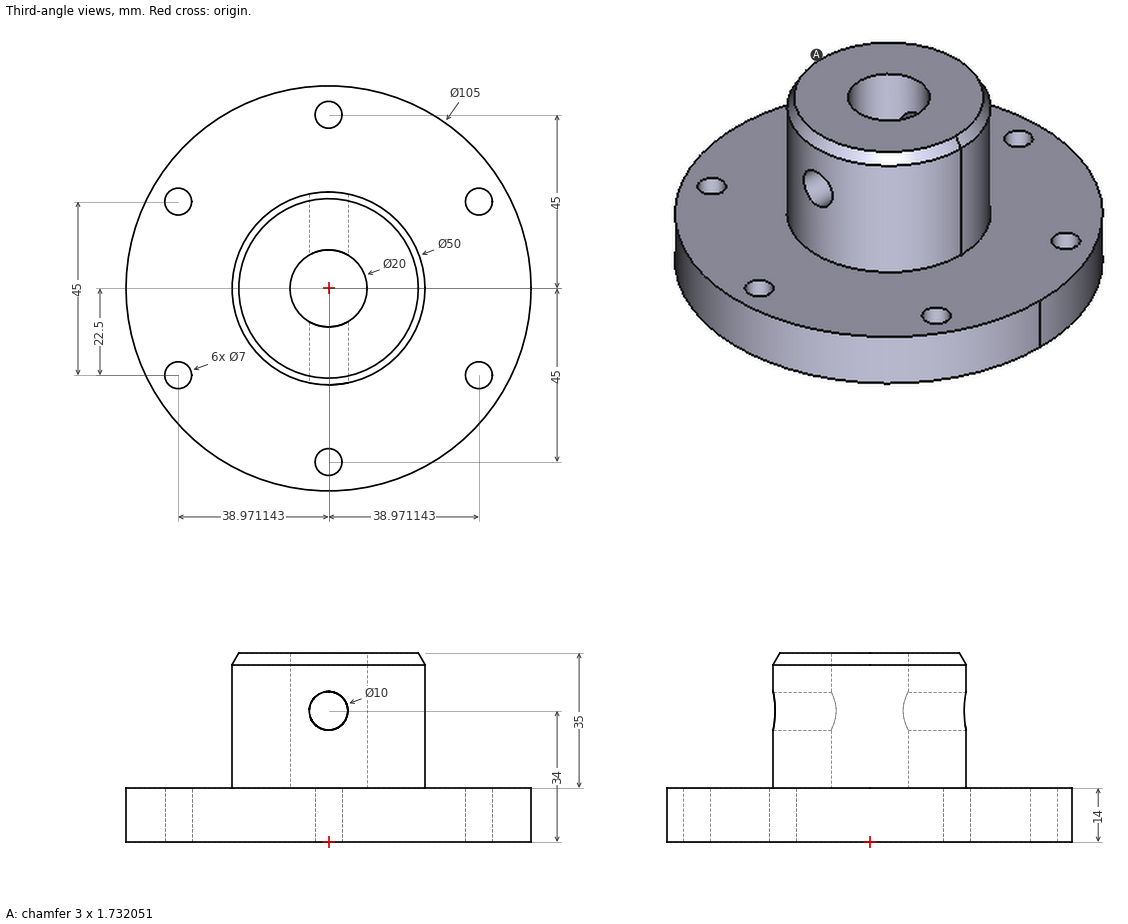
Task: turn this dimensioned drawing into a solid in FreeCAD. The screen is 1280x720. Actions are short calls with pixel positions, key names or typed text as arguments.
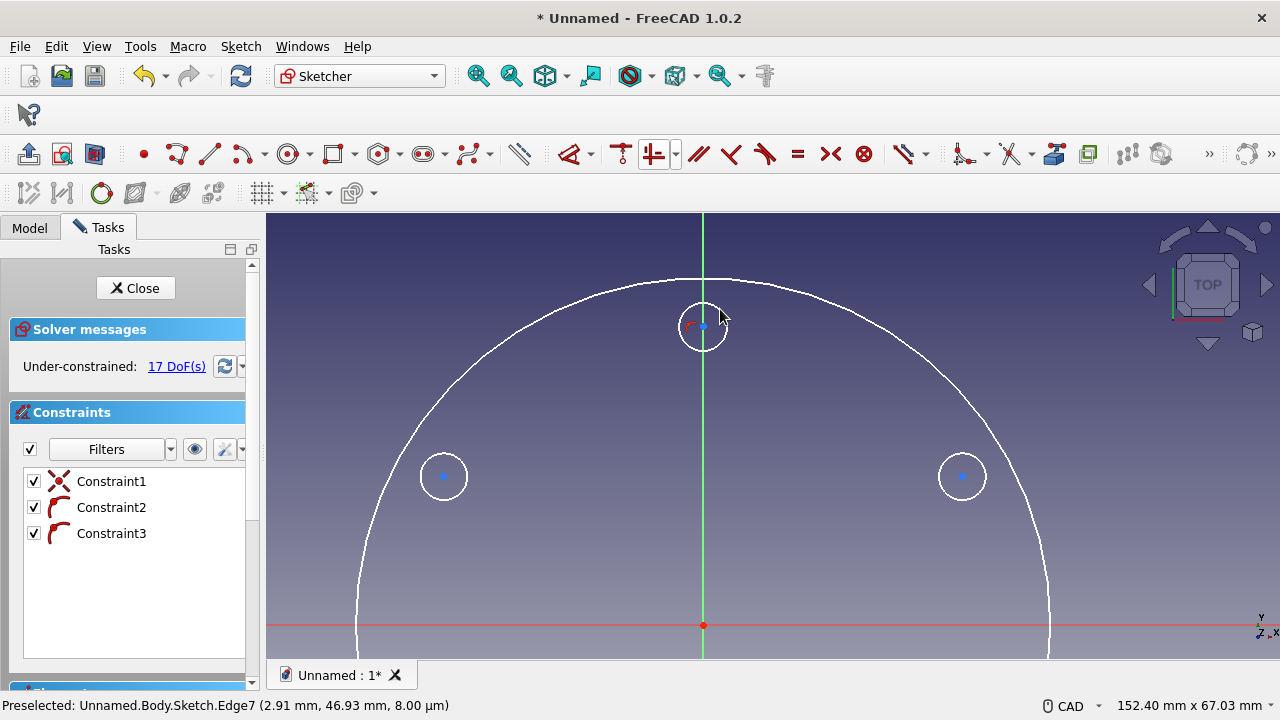
scroll(705, 326, down, 5)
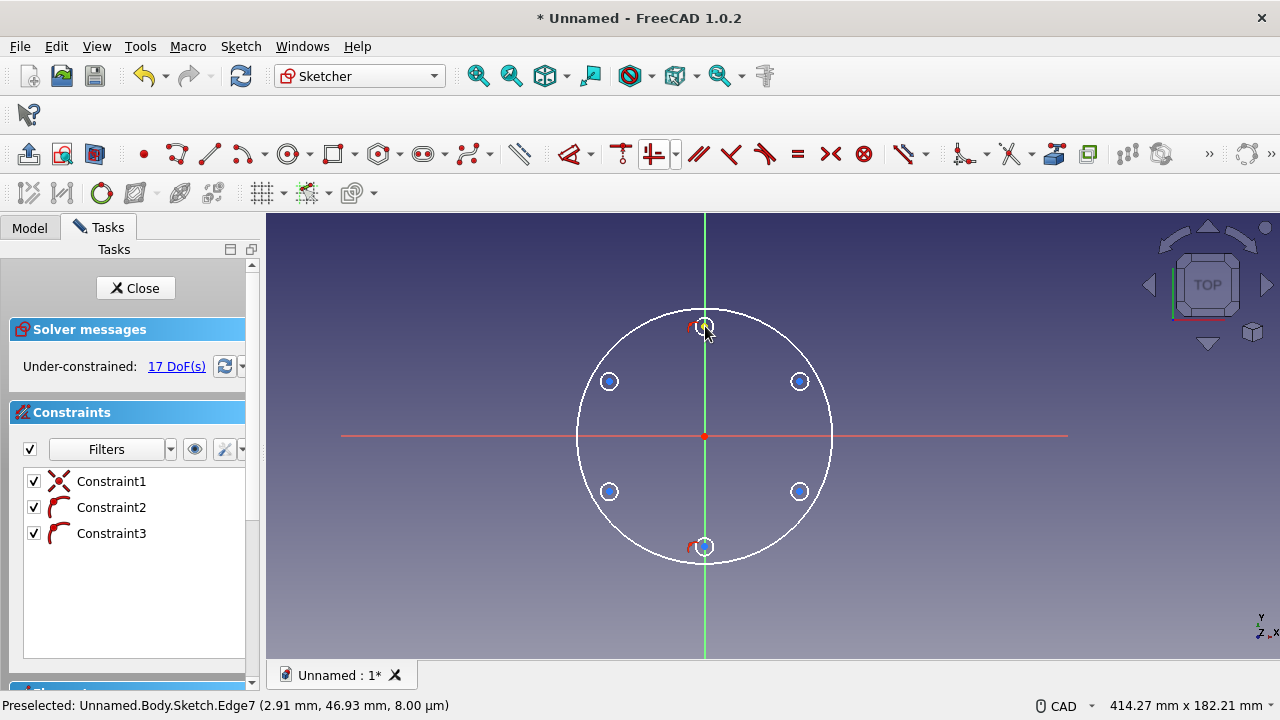
scroll(615, 486, up, 3)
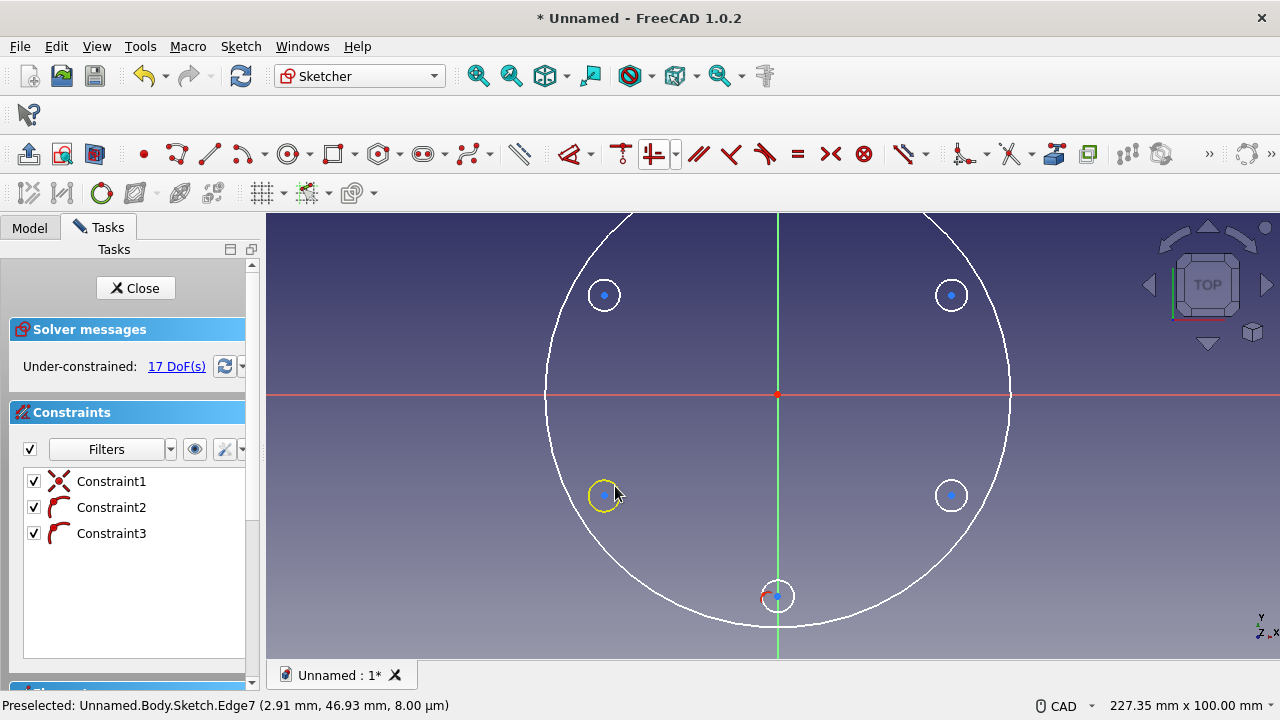
click(615, 485)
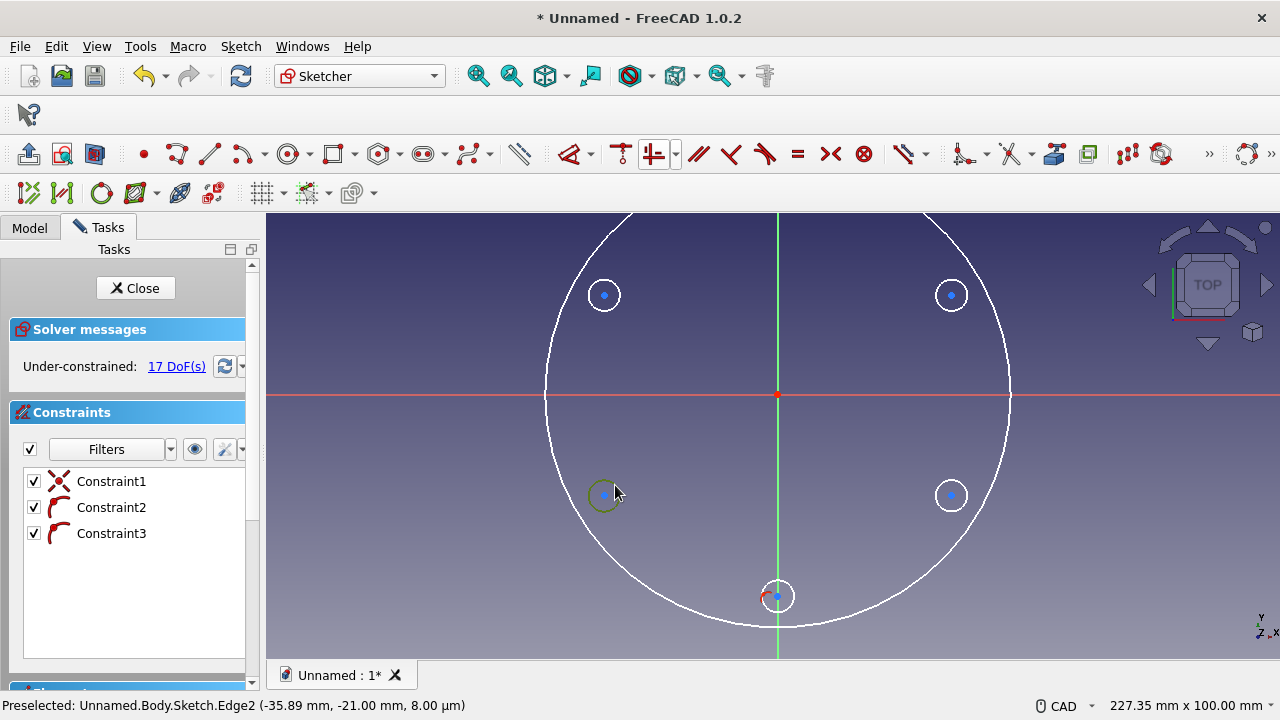
click(789, 585)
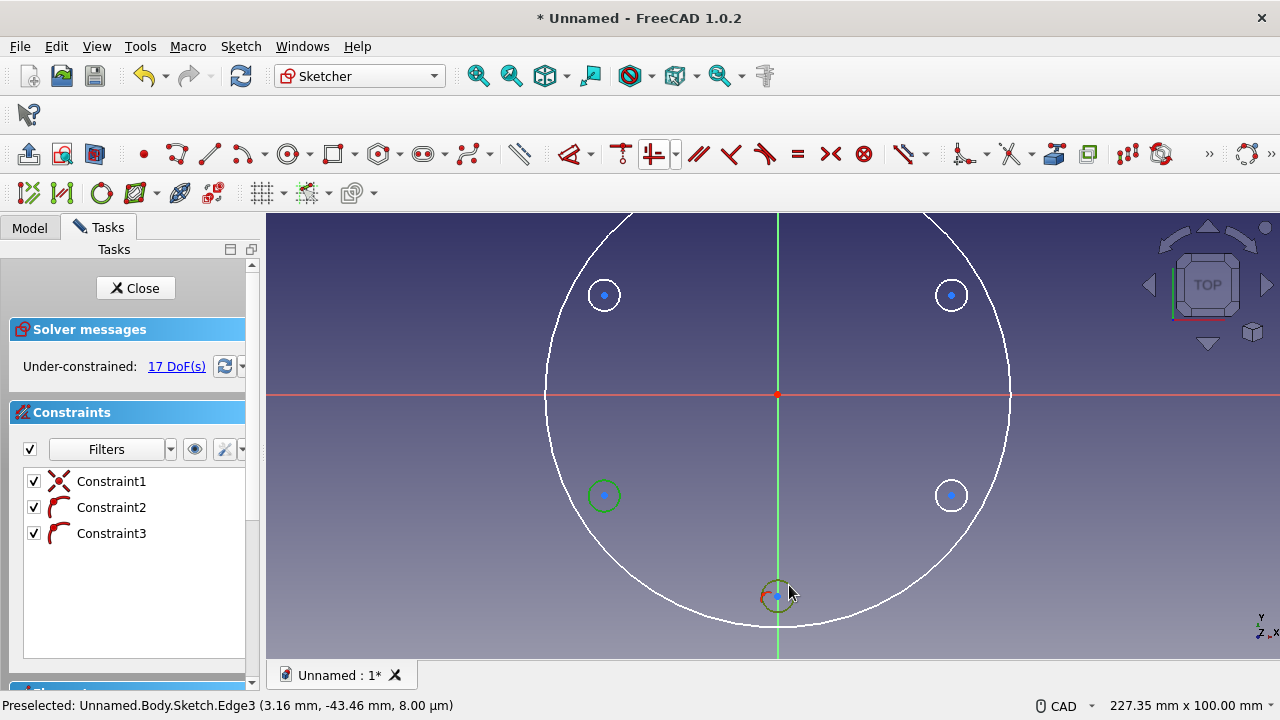
click(963, 485)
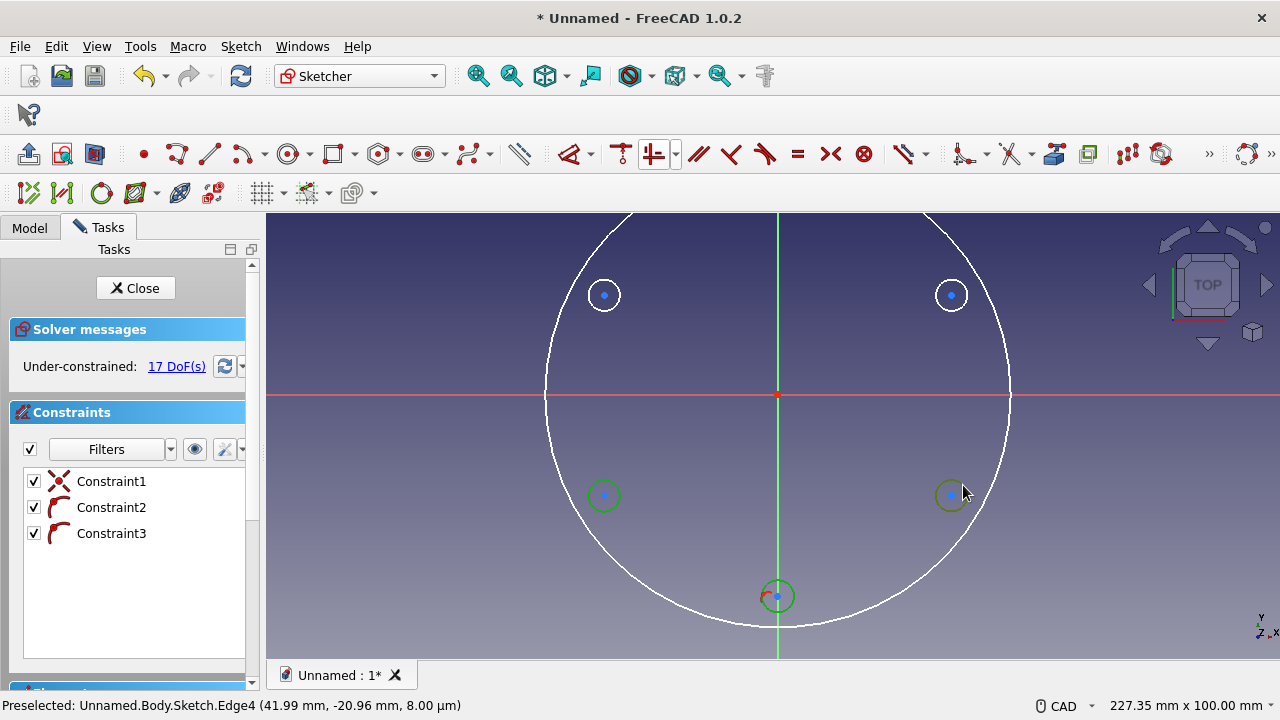
click(615, 284)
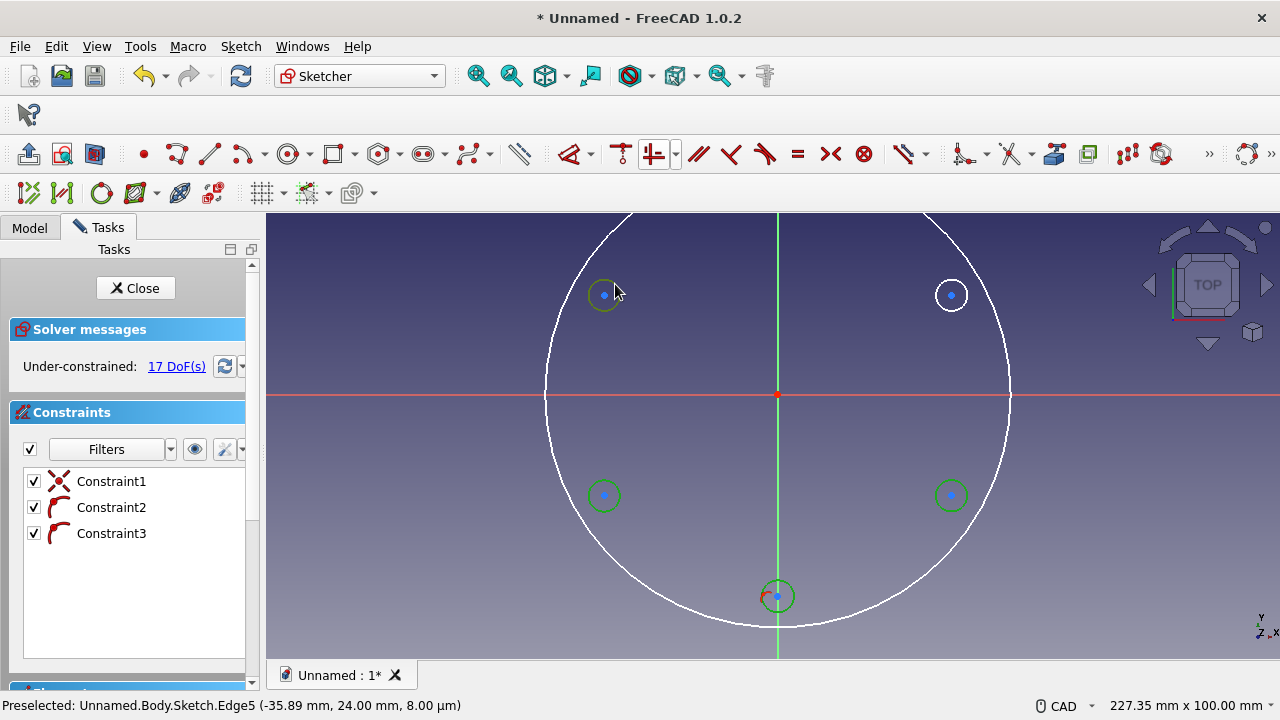
click(963, 284)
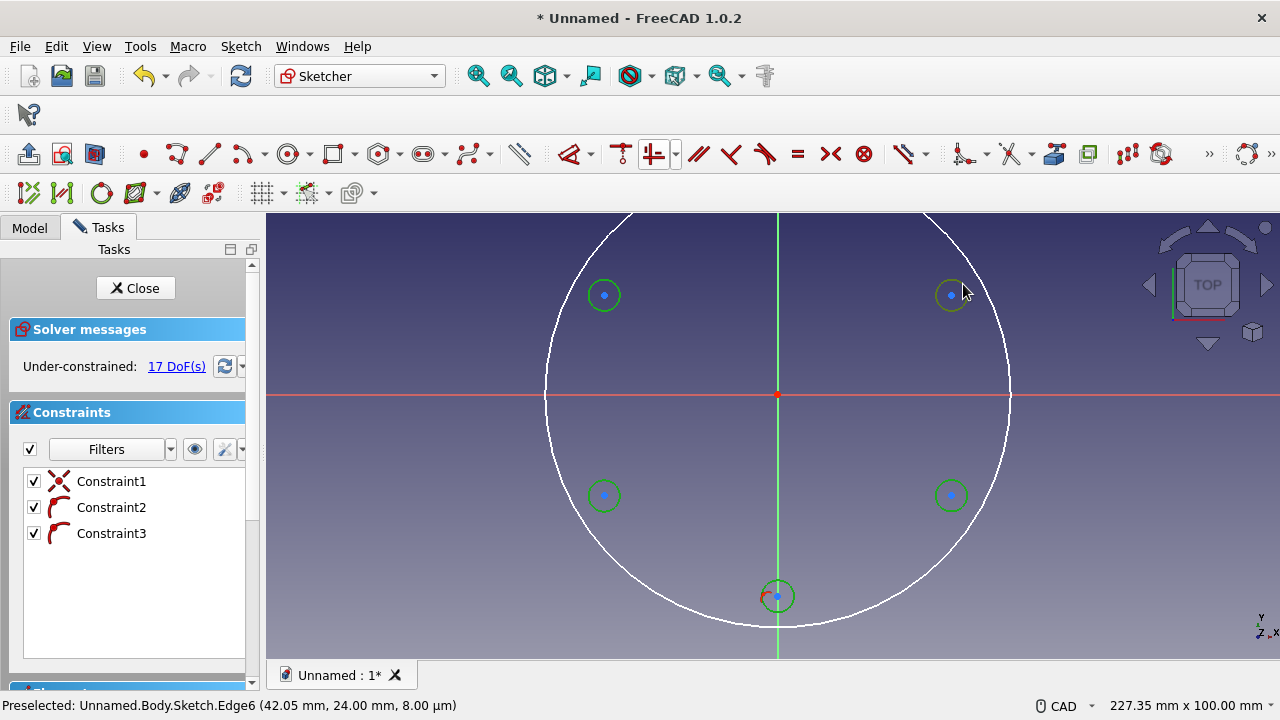
scroll(615, 486, down, 3)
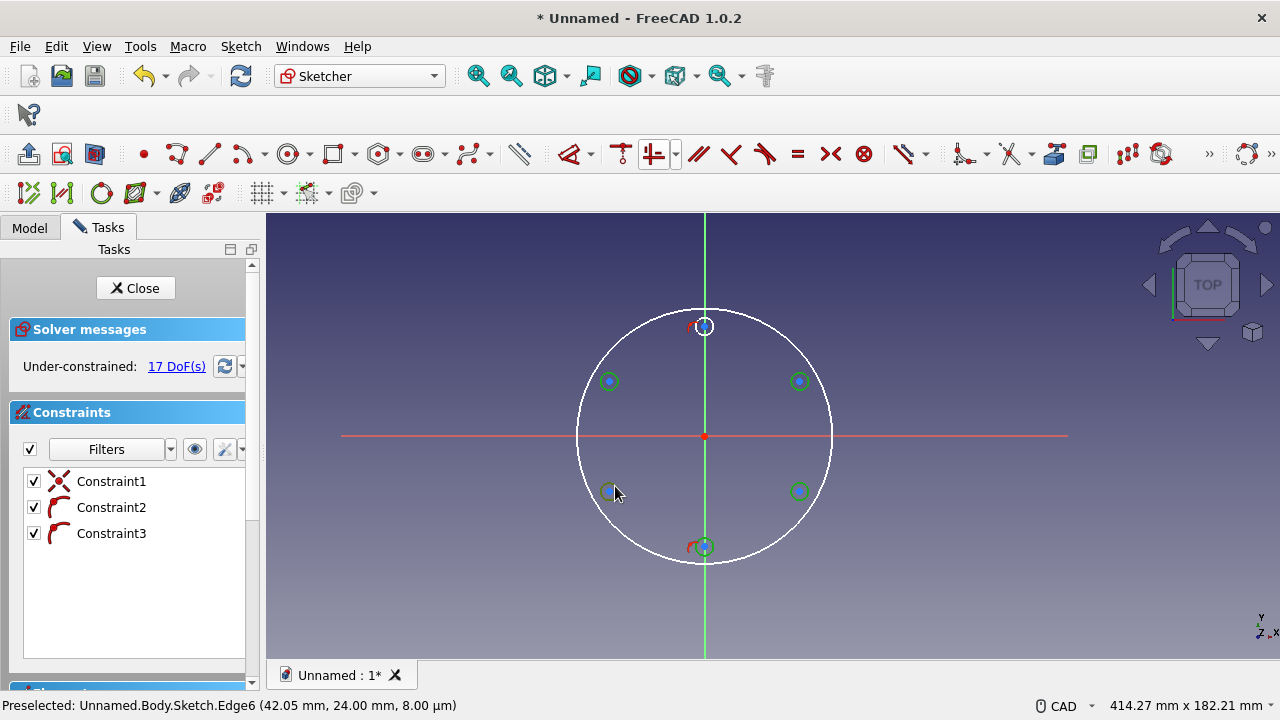
scroll(711, 320, up, 4)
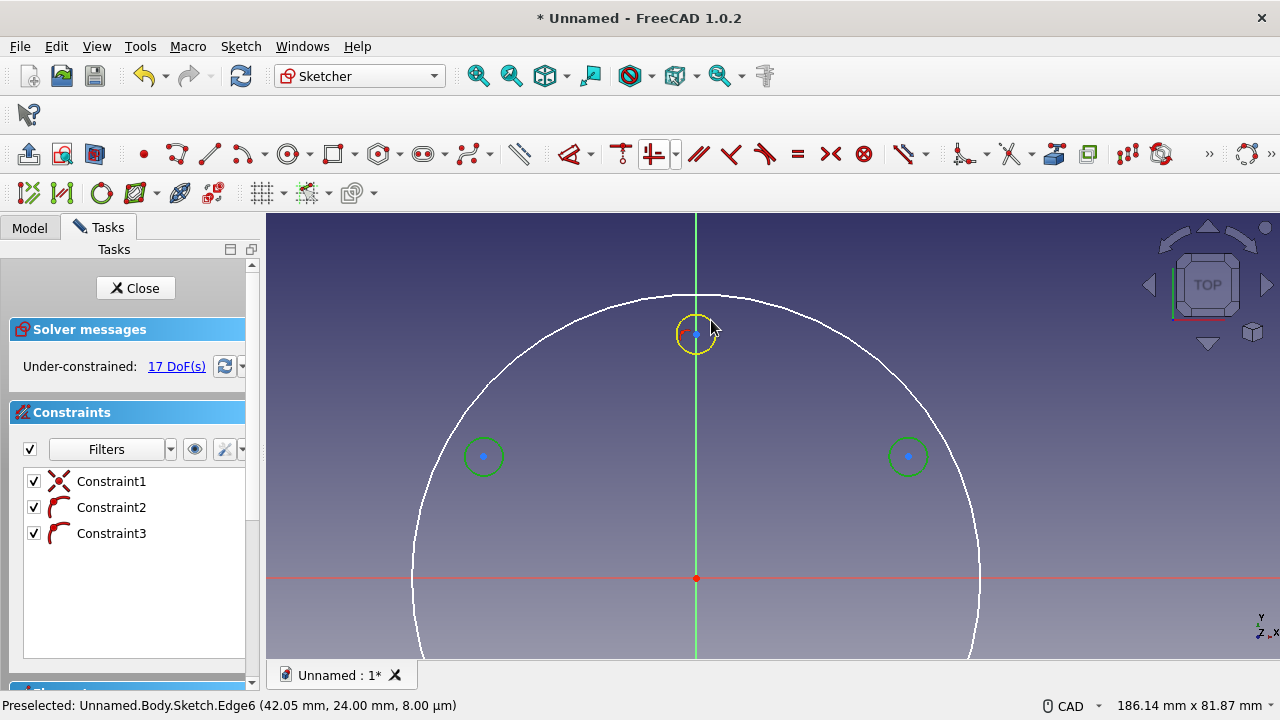
click(710, 320)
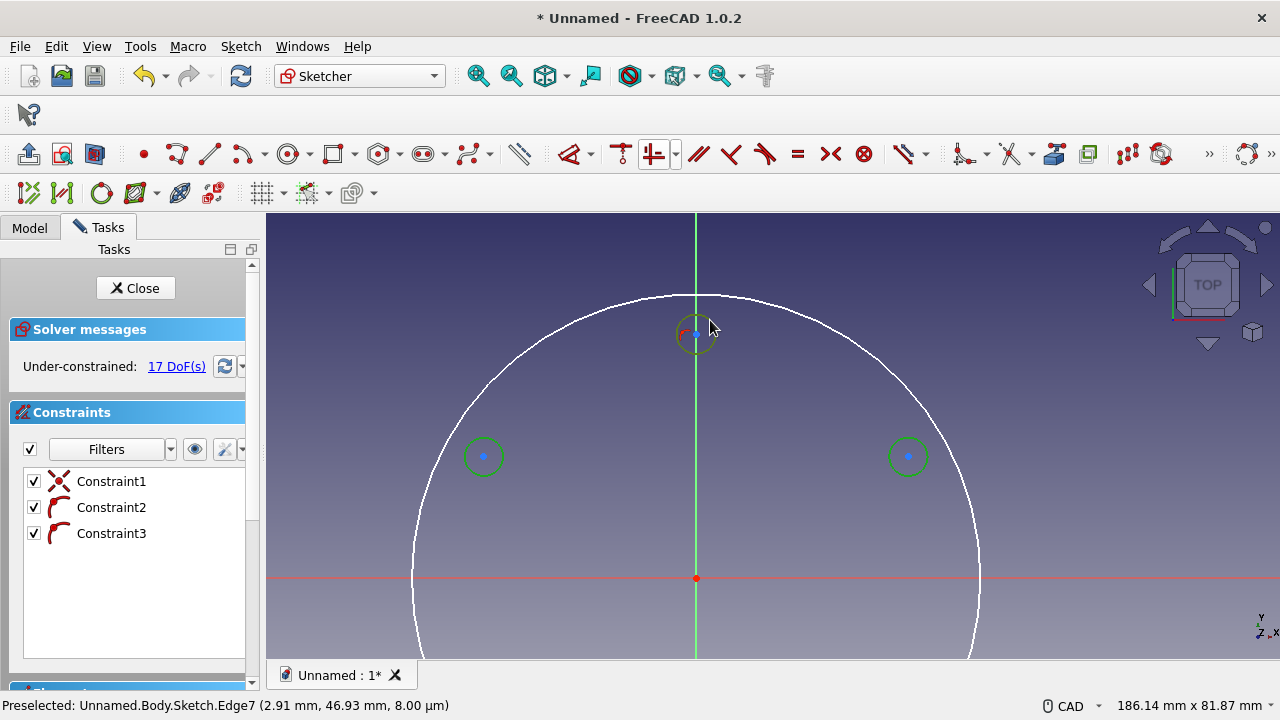
click(798, 154)